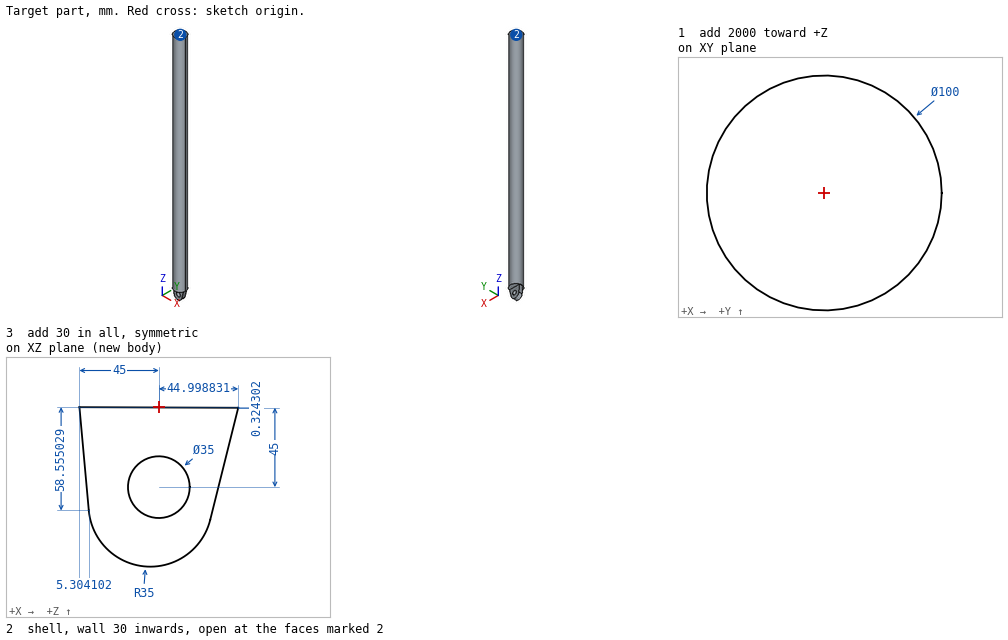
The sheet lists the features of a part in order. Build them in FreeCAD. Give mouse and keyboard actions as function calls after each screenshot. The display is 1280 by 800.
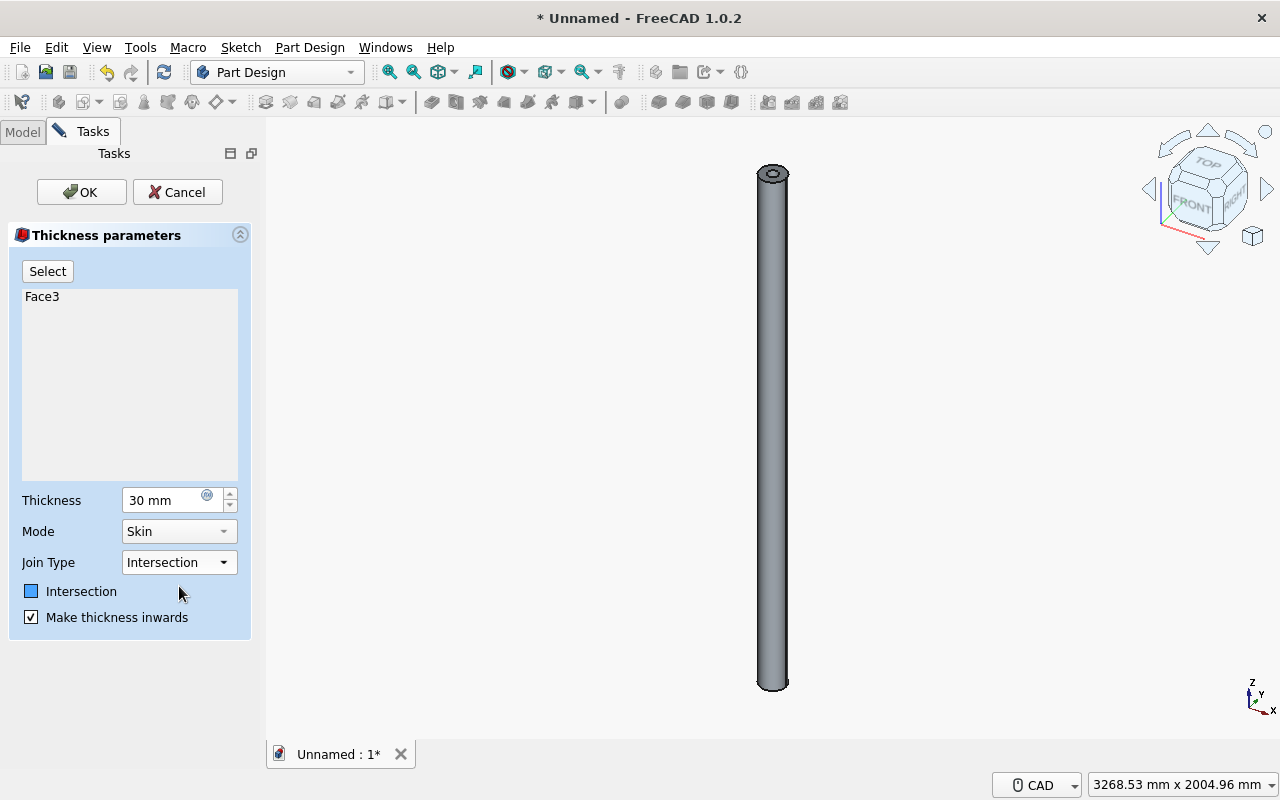
click(82, 192)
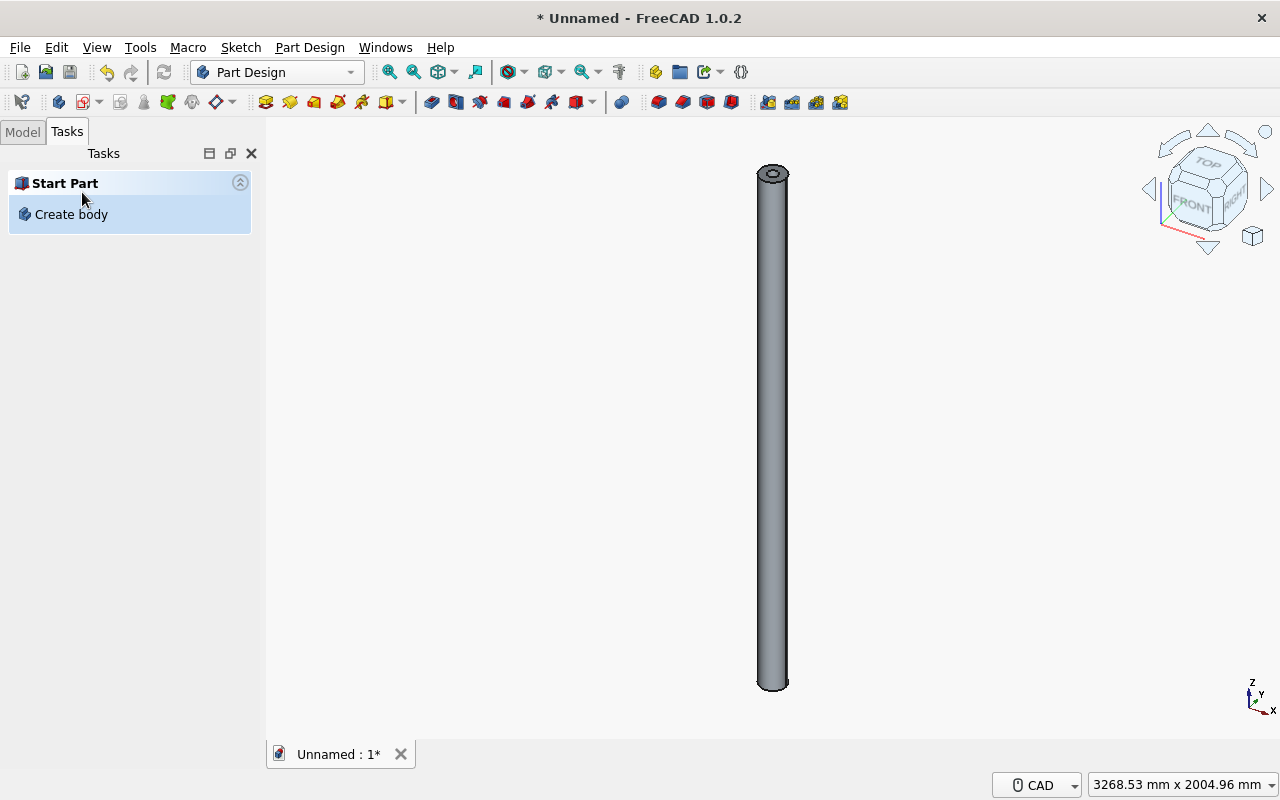
click(60, 102)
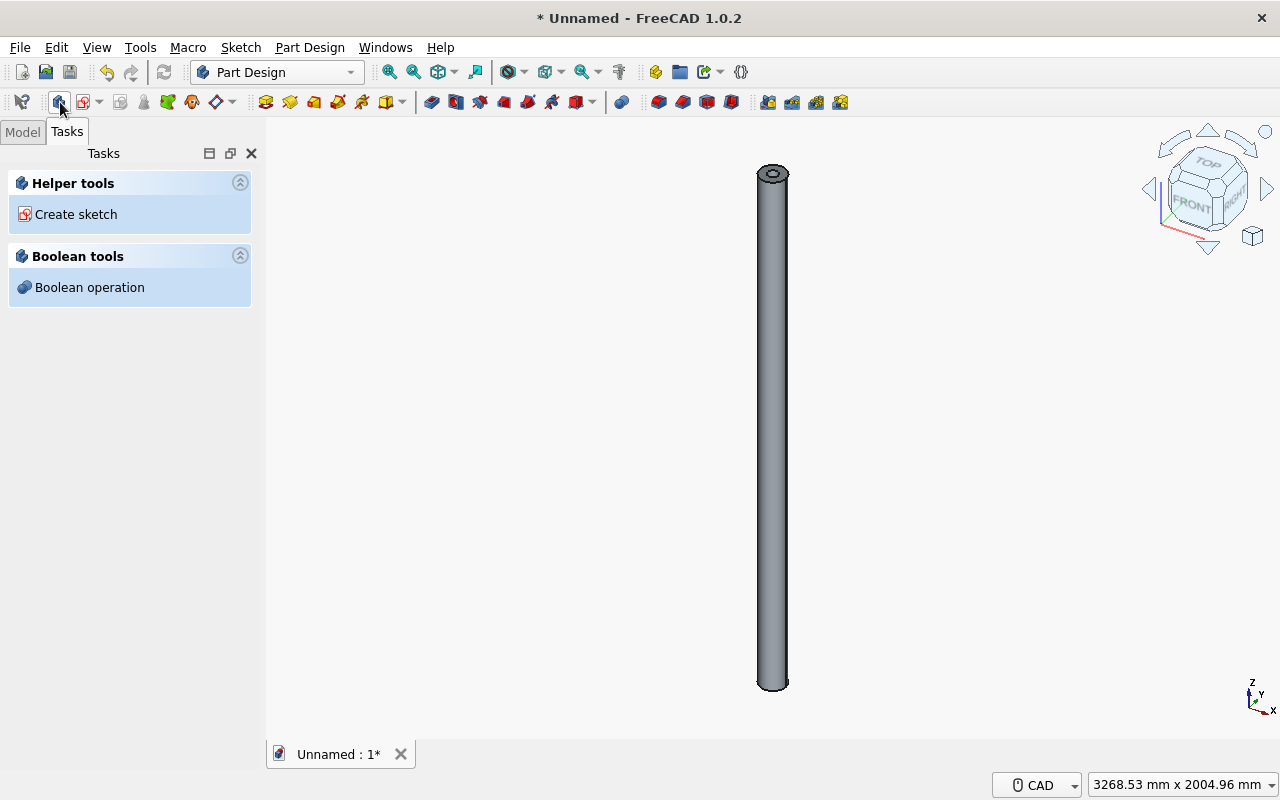
click(306, 699)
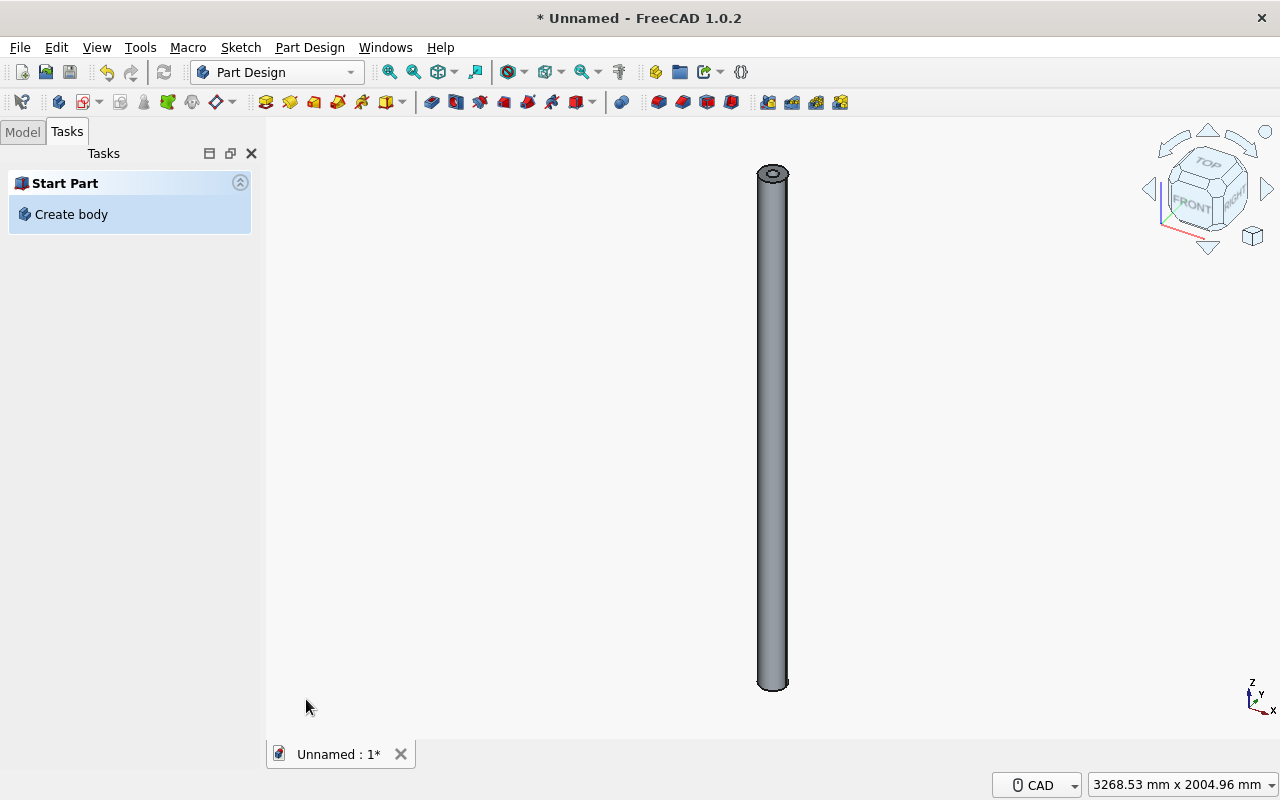
click(84, 102)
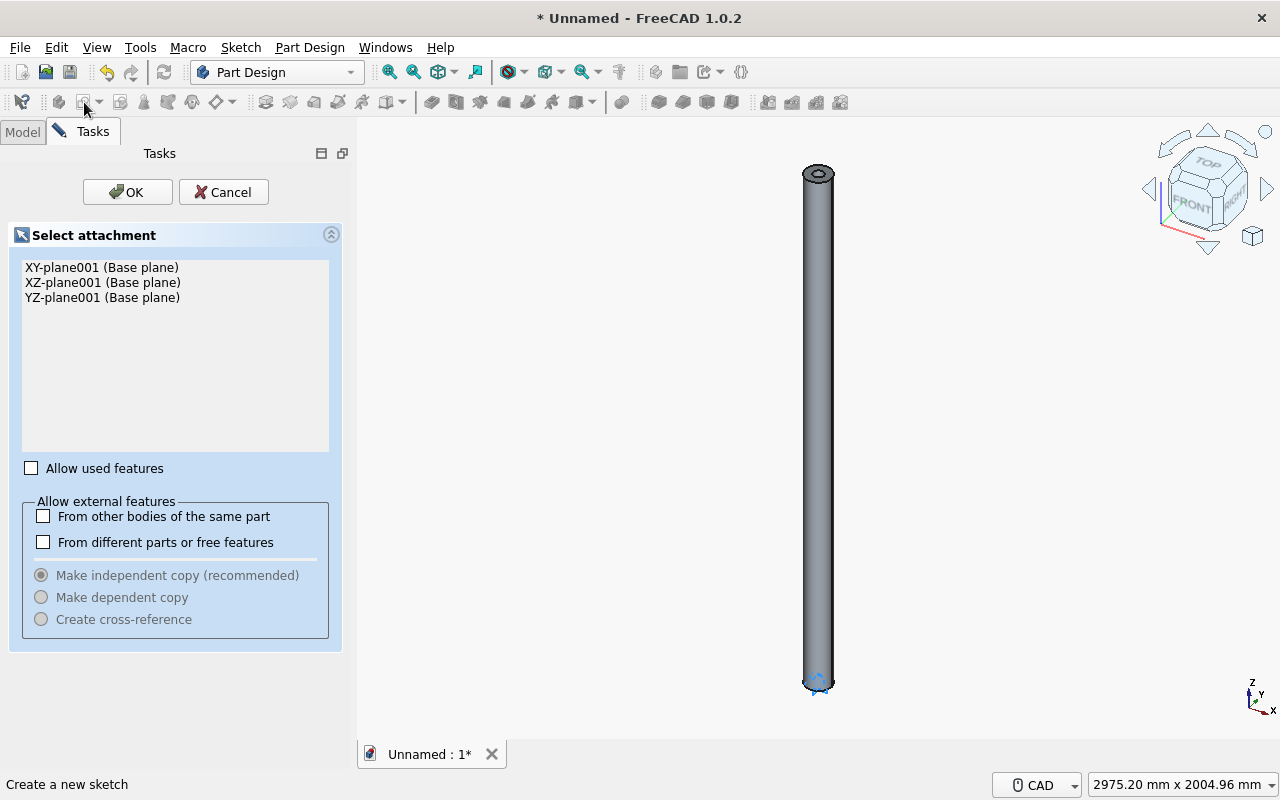
click(82, 282)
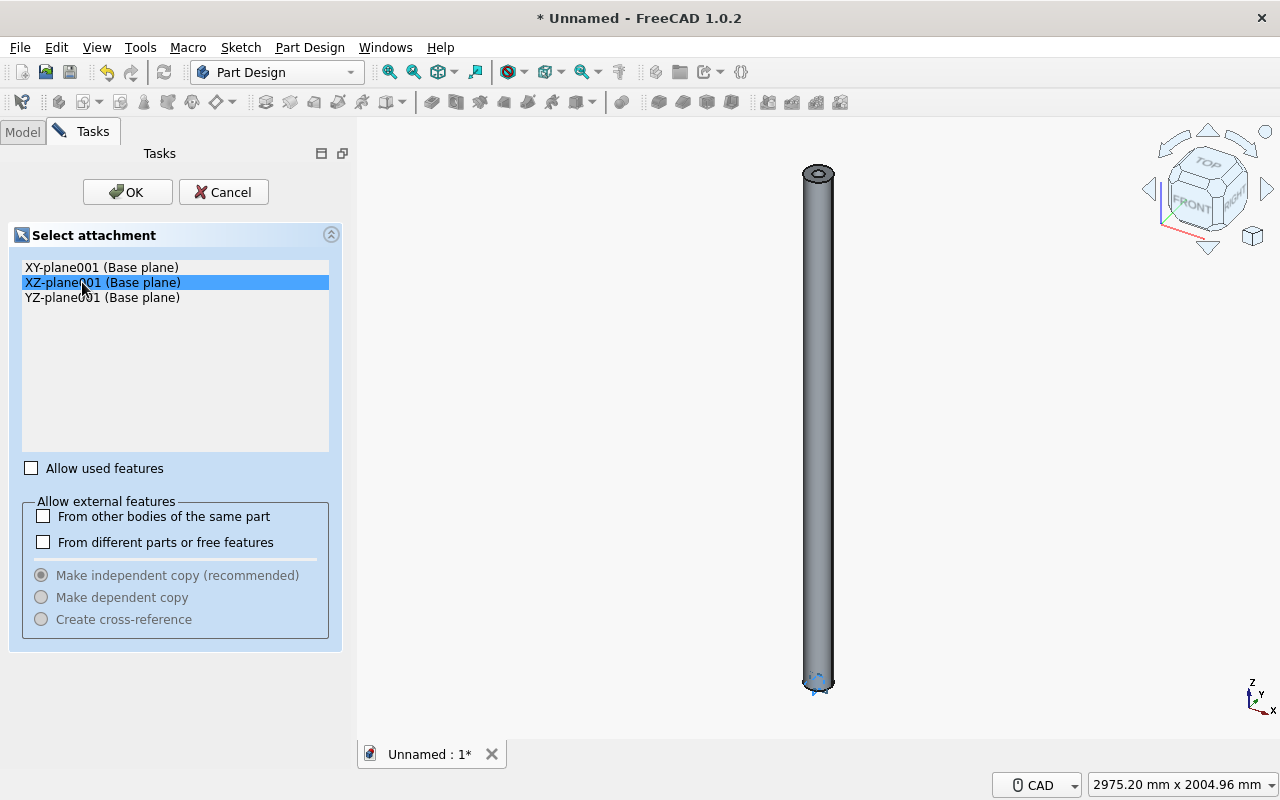
click(128, 192)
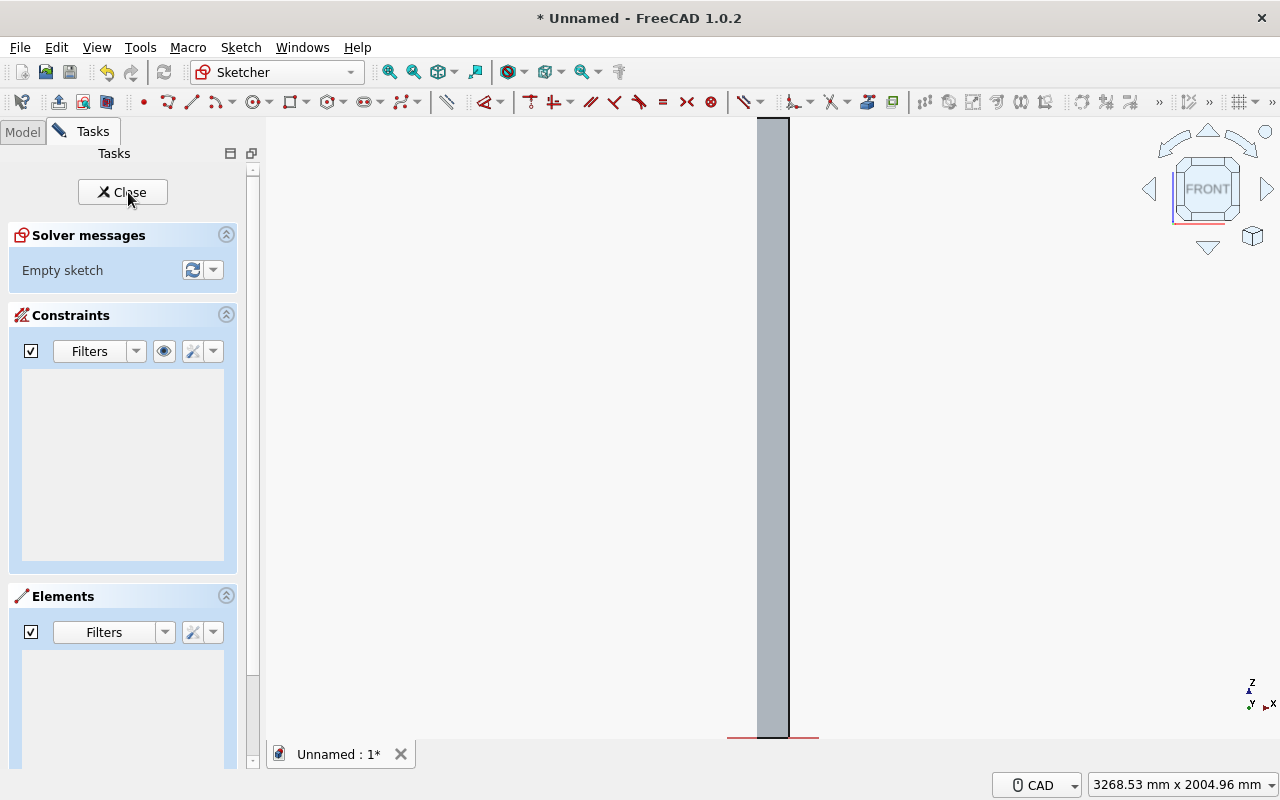
scroll(704, 428, down, 5)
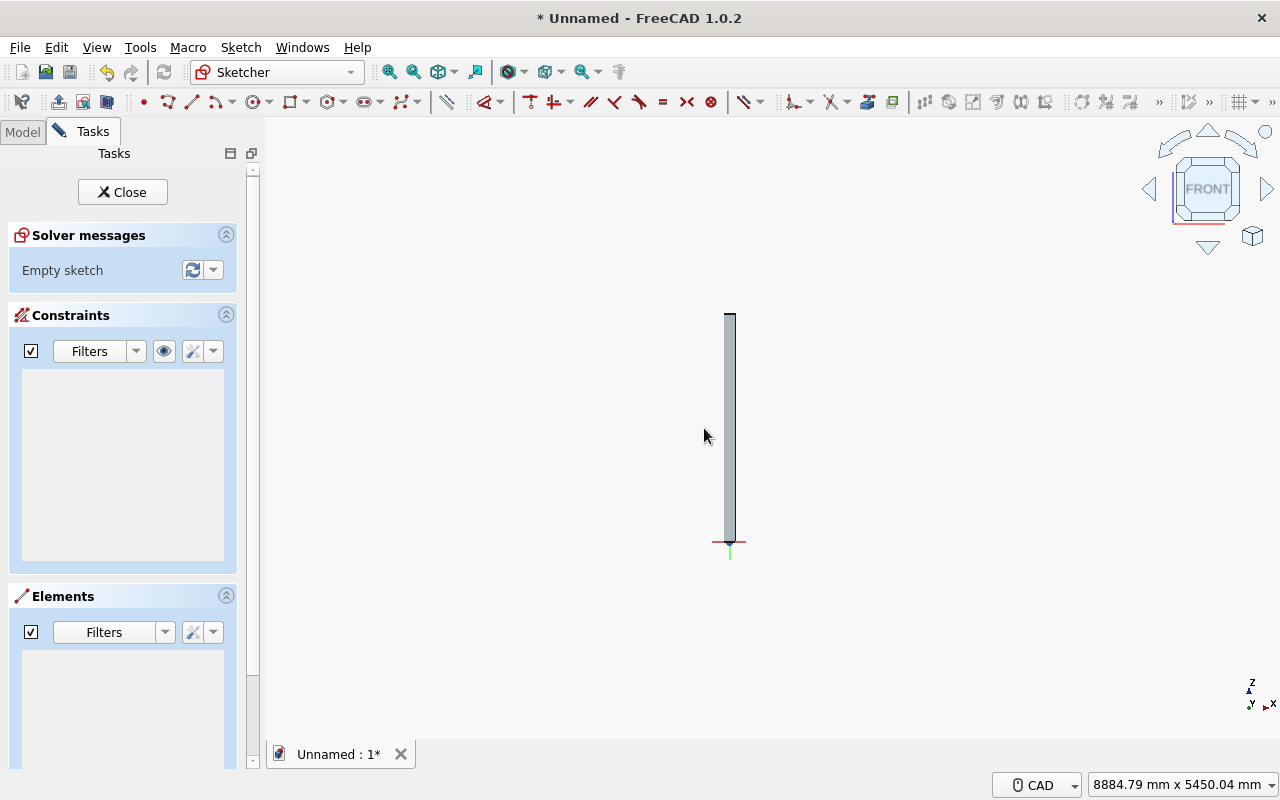
scroll(731, 554, up, 15)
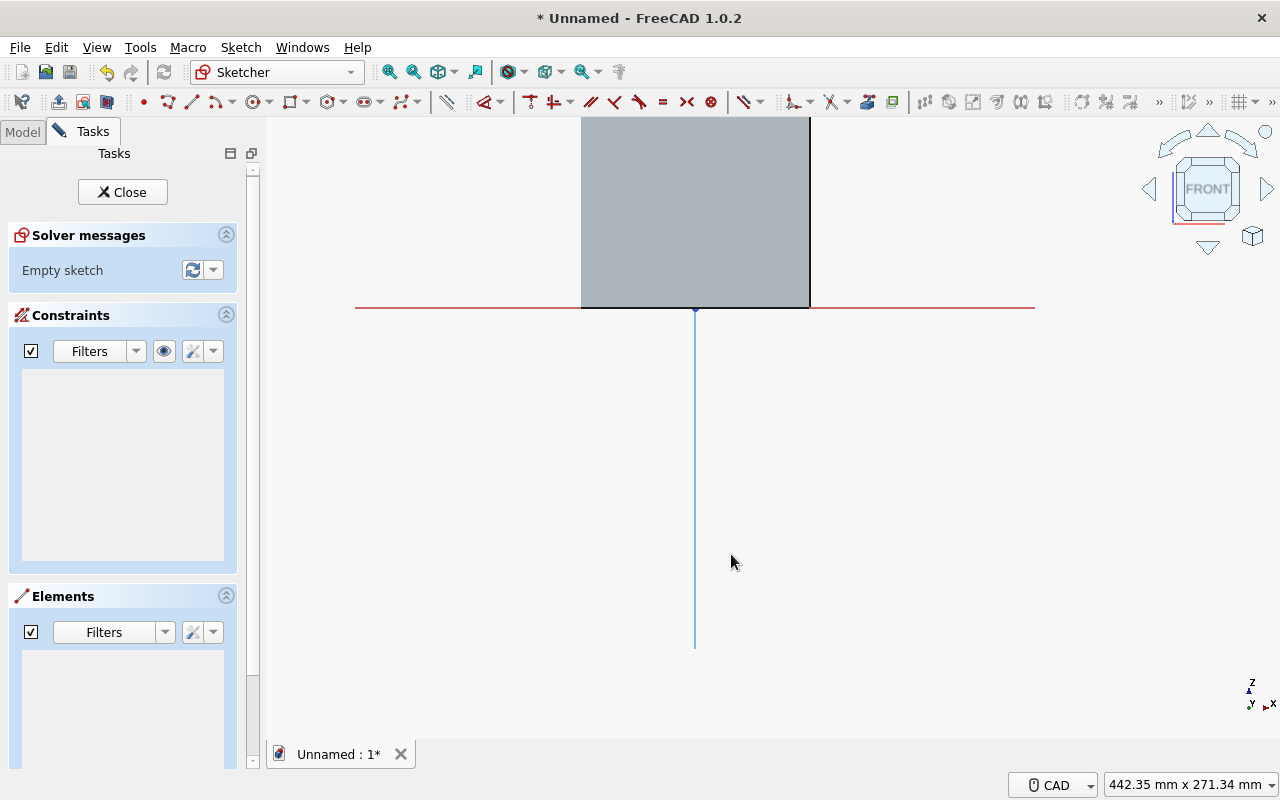
scroll(684, 392, up, 3)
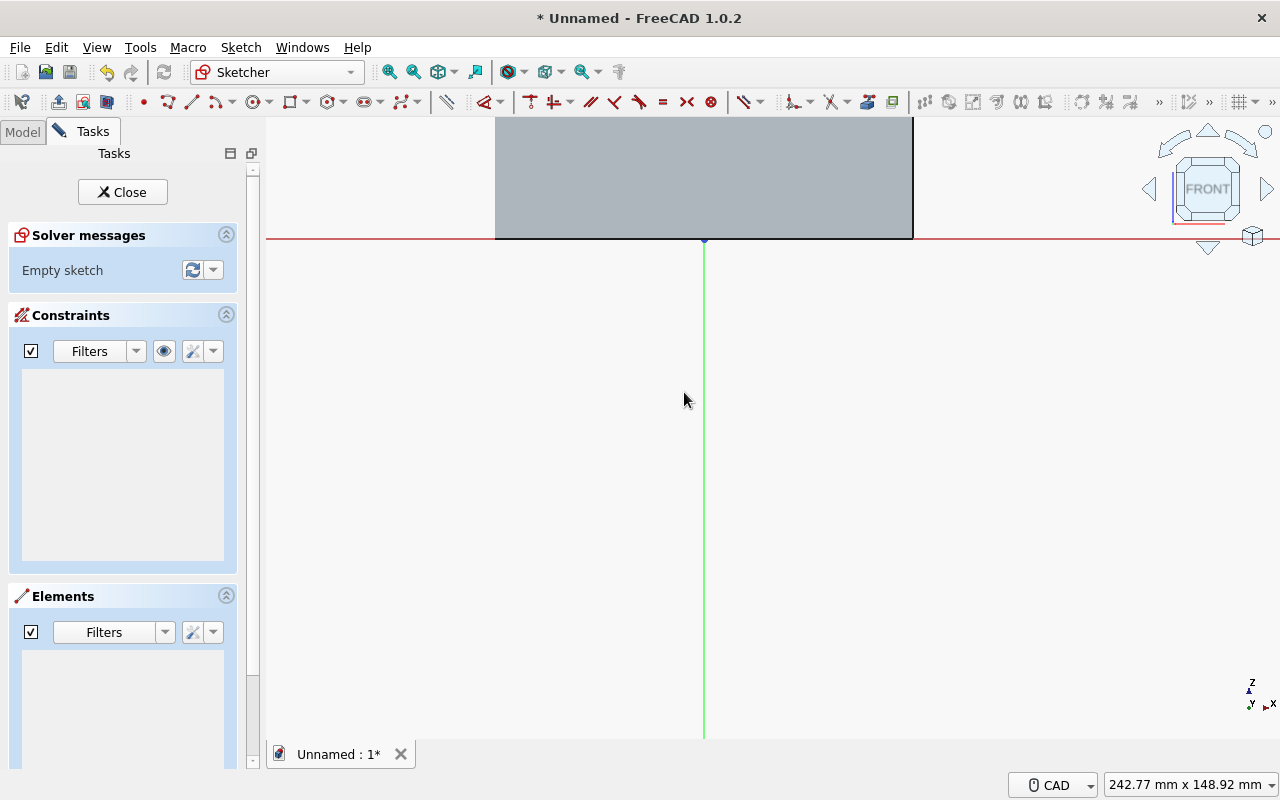
key(g)
key(m)